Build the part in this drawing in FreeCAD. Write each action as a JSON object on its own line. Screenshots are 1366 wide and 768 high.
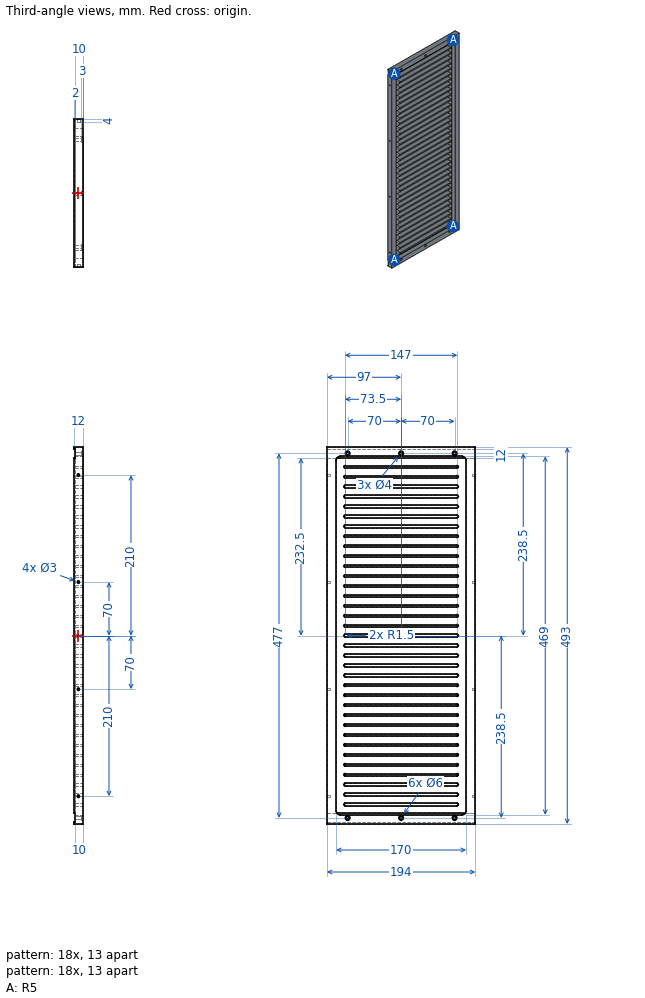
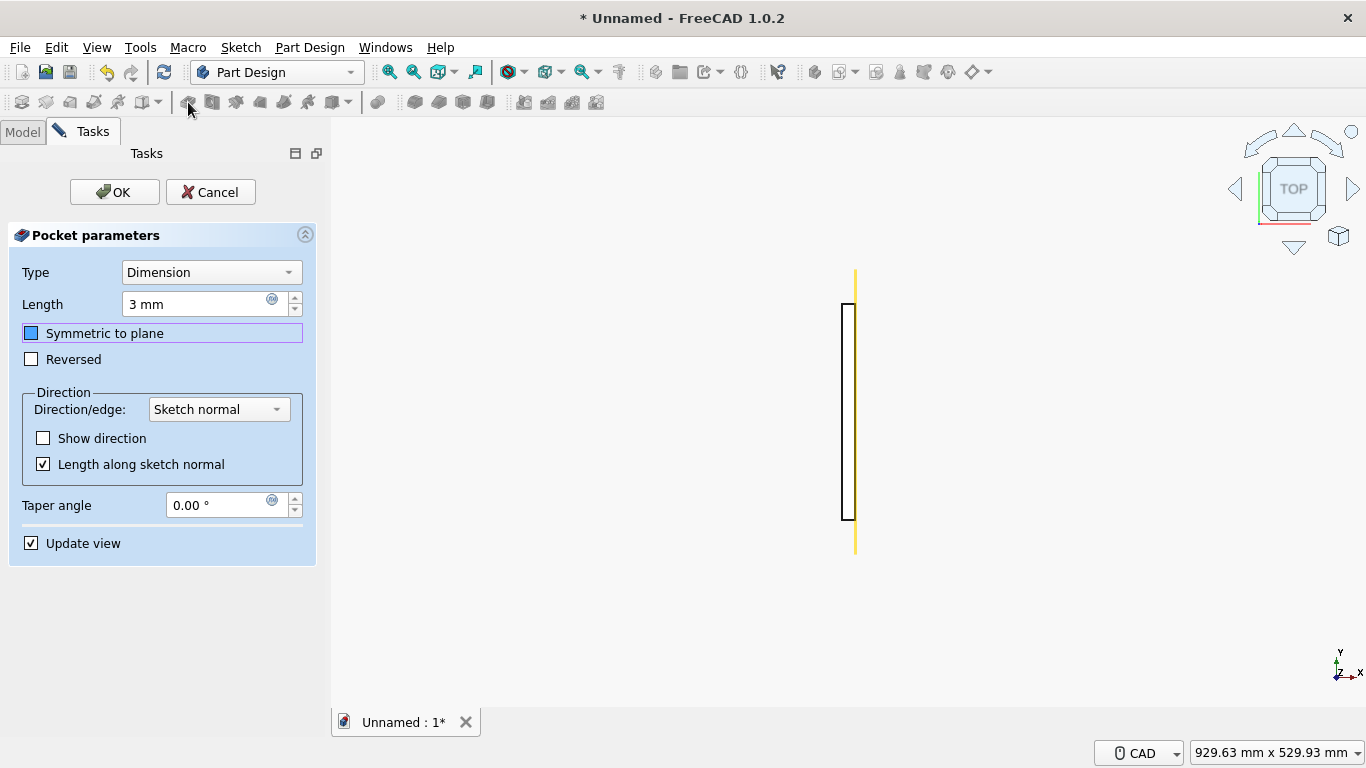
{"action": "left_click", "coordinate": [115, 192]}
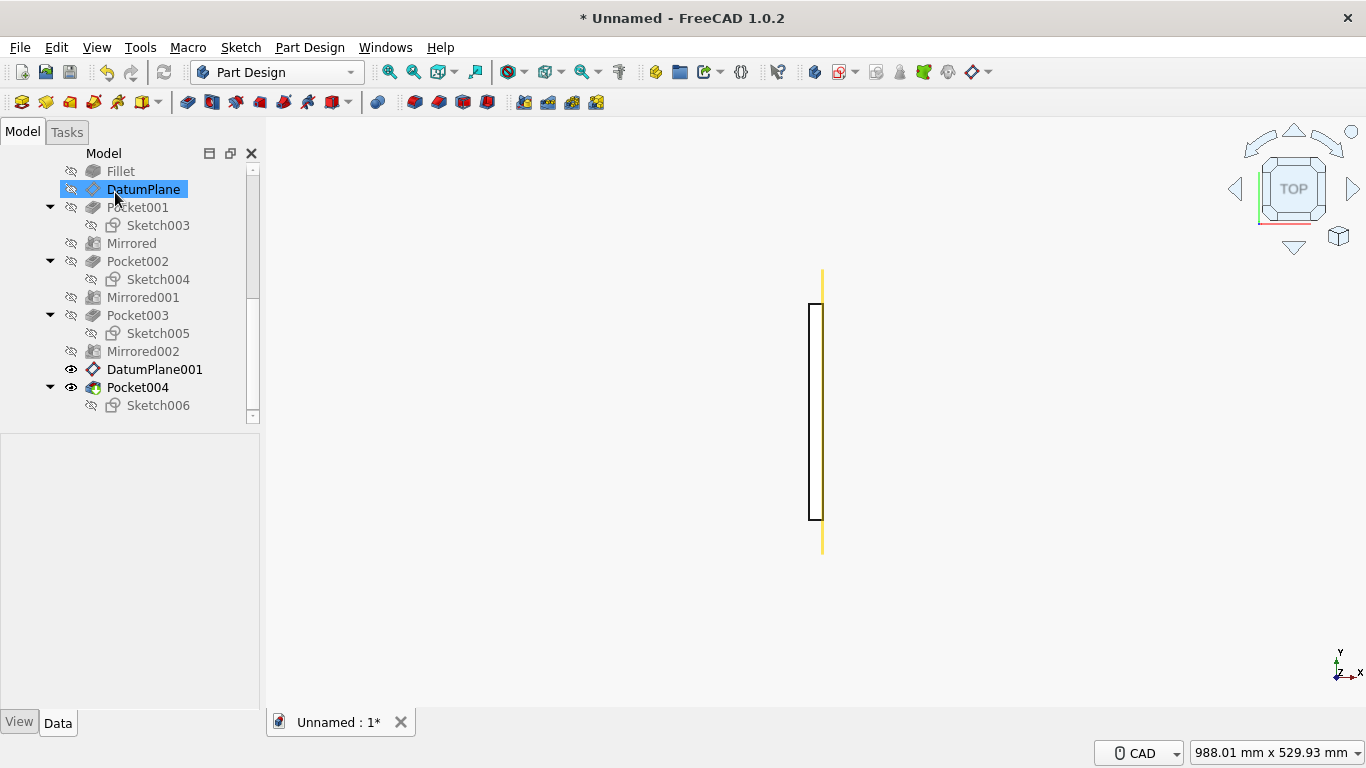
{"action": "left_click", "coordinate": [116, 369]}
{"action": "key", "text": "space"}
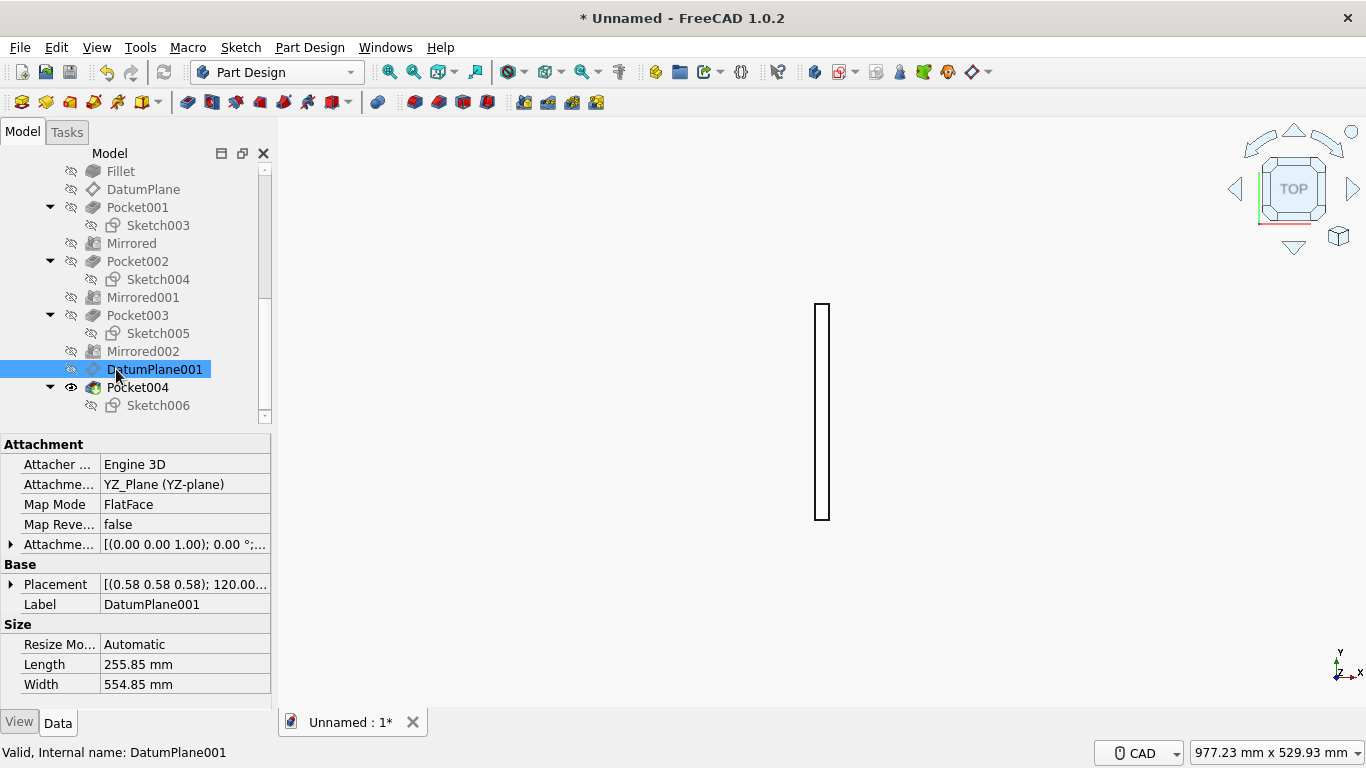
{"action": "key", "text": "0"}